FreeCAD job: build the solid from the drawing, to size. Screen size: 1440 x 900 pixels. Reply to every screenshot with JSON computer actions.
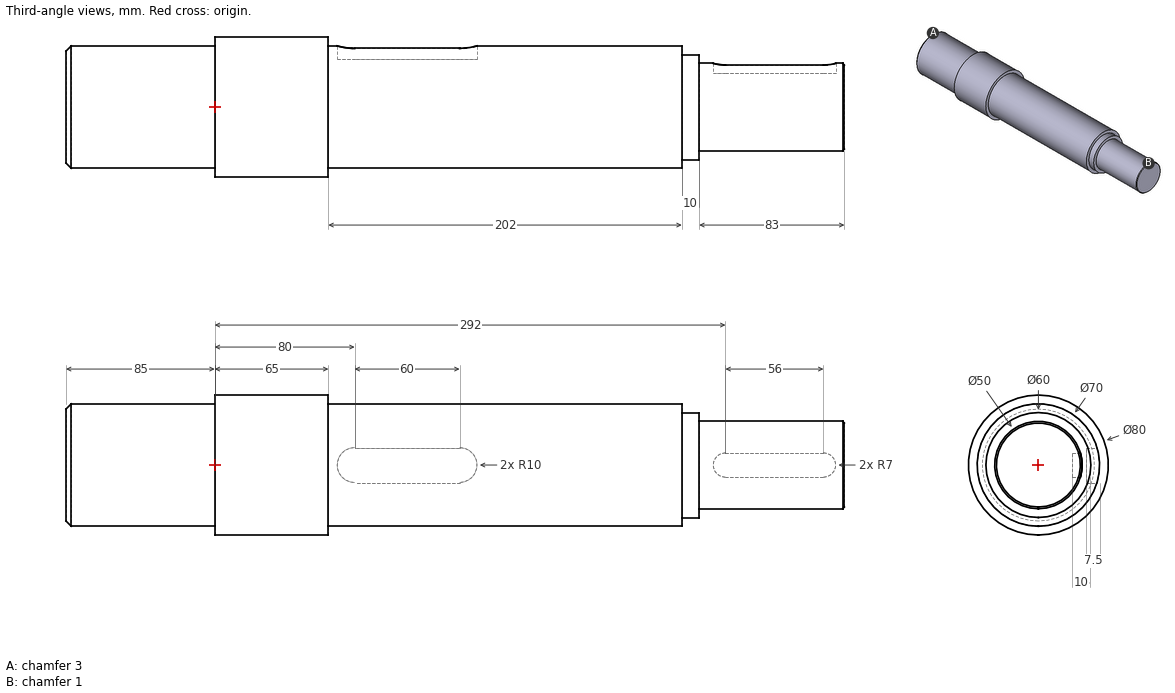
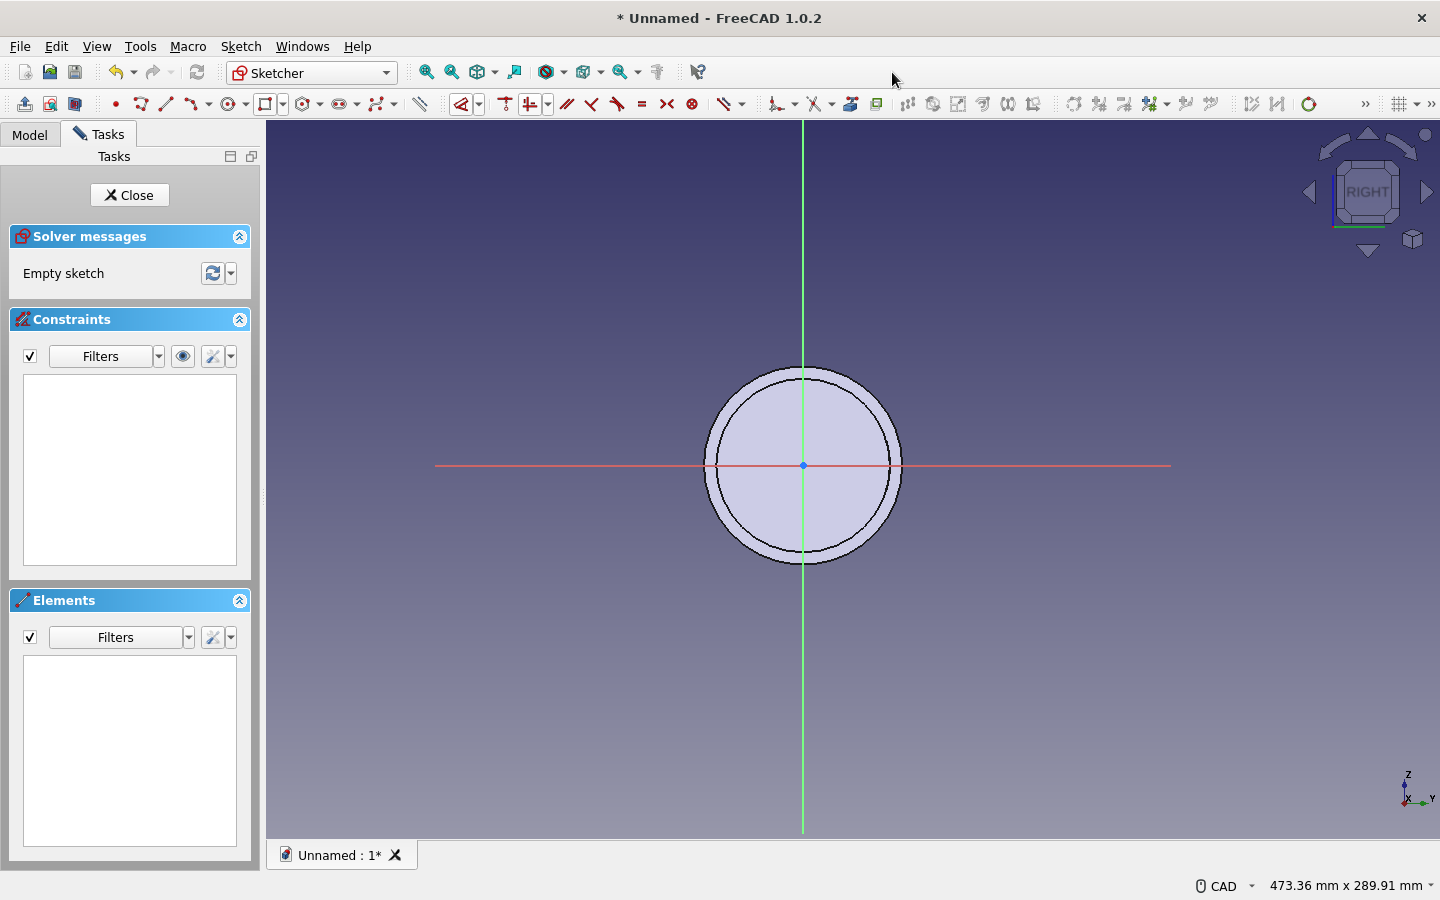
{"action": "scroll", "coordinate": [811, 460], "scroll_direction": "up", "scroll_amount": 6}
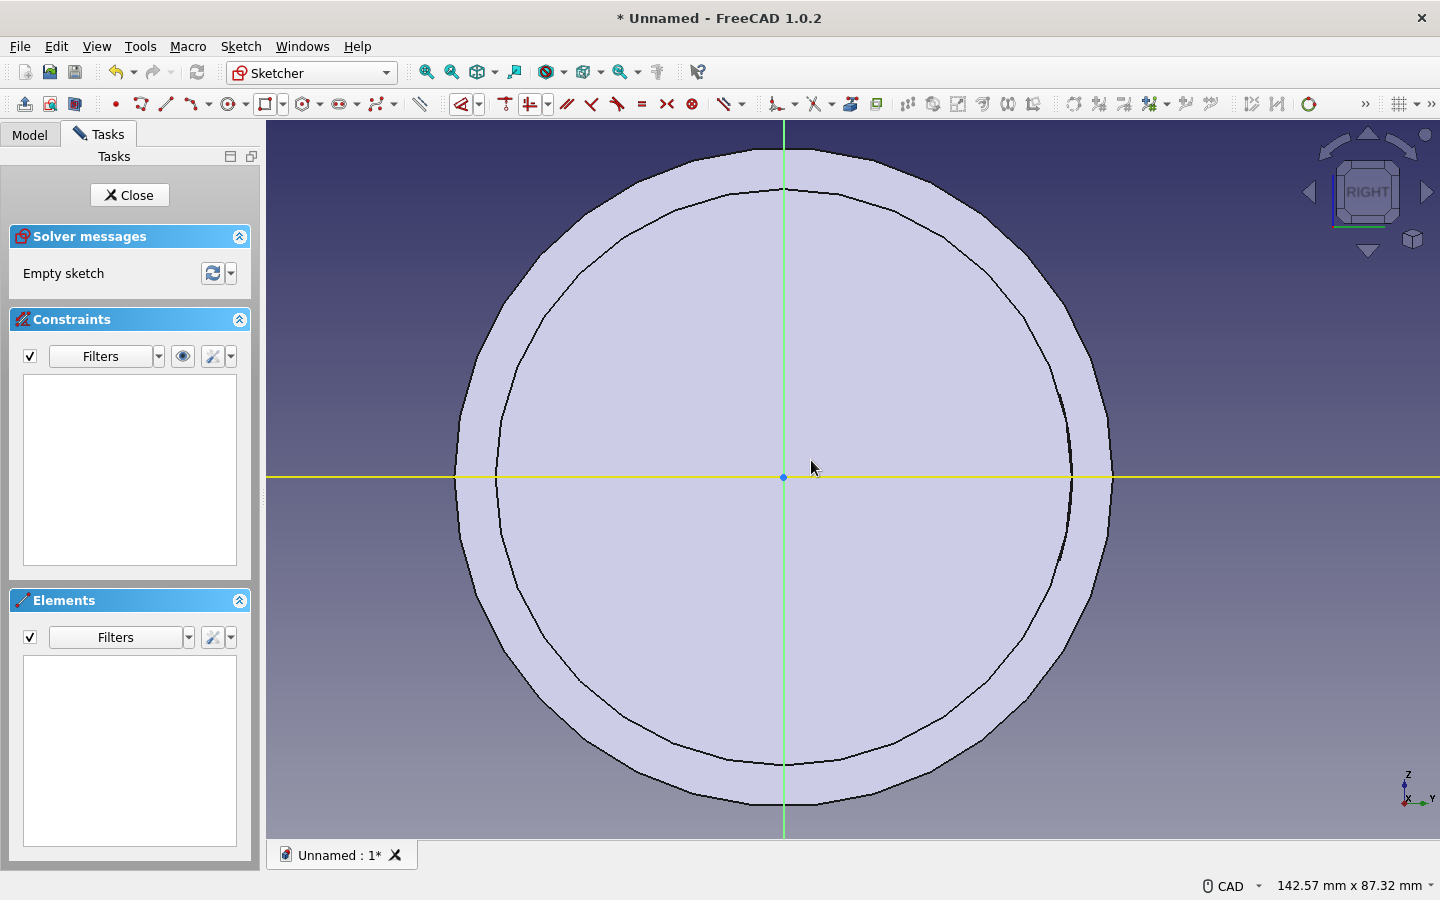
{"action": "key", "text": "g c"}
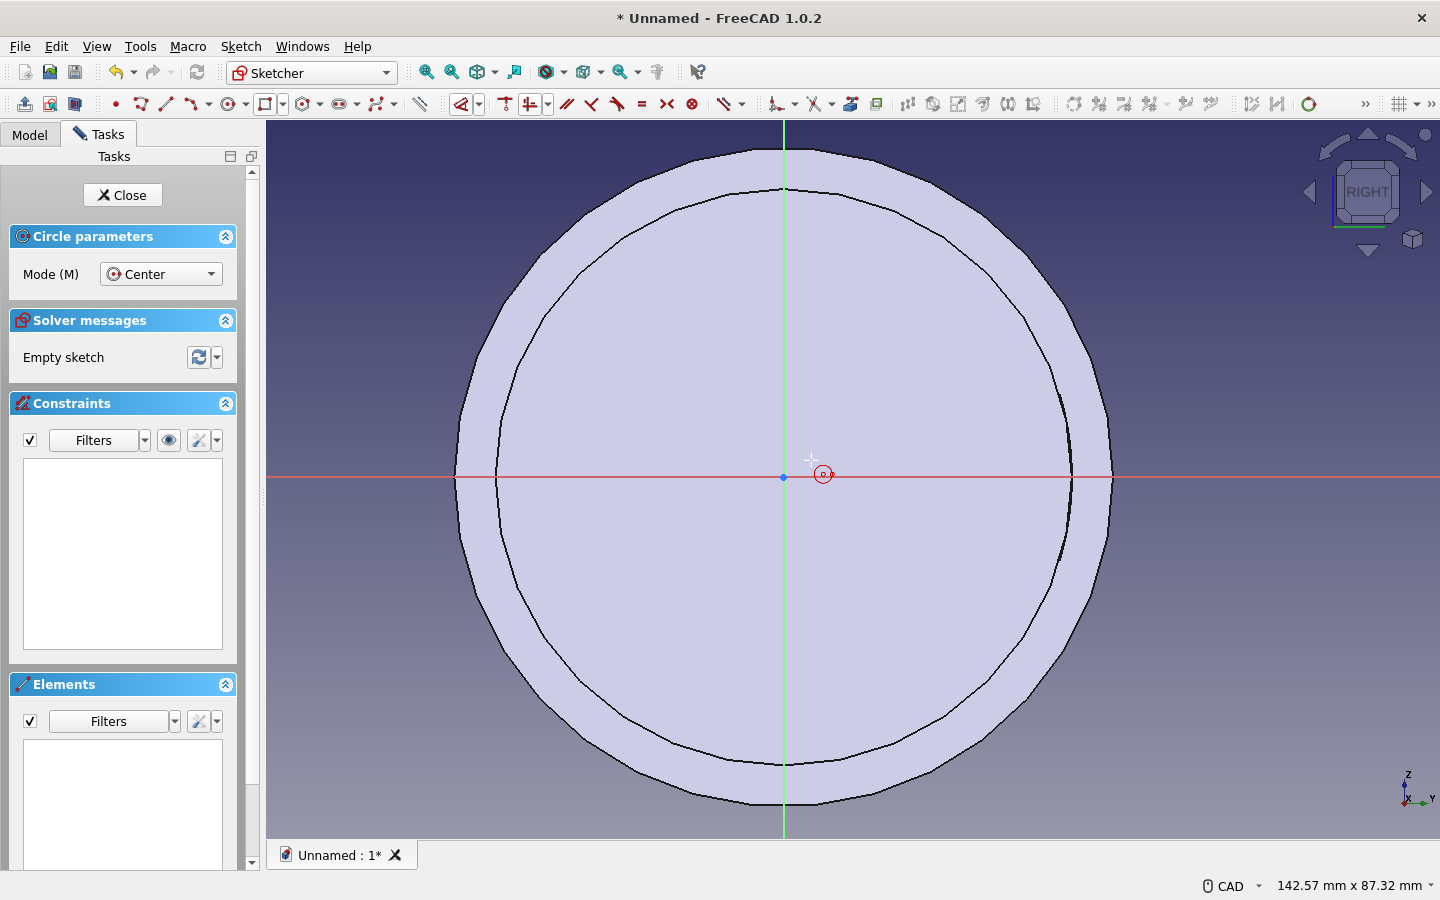
{"action": "left_click", "coordinate": [784, 477]}
{"action": "left_click", "coordinate": [958, 303]}
{"action": "key", "text": "Escape"}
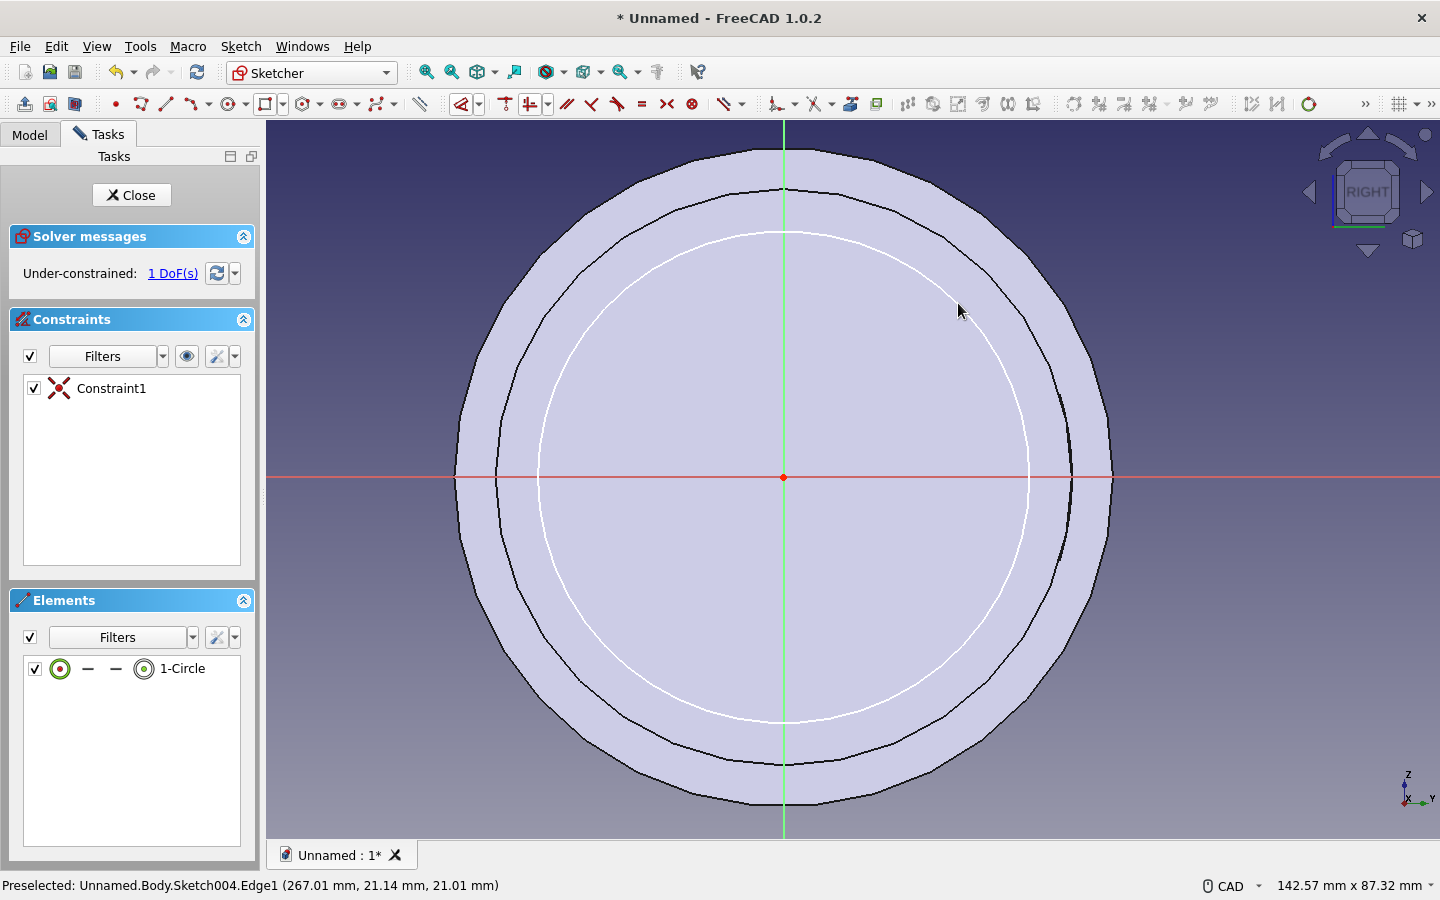
{"action": "left_click", "coordinate": [460, 104]}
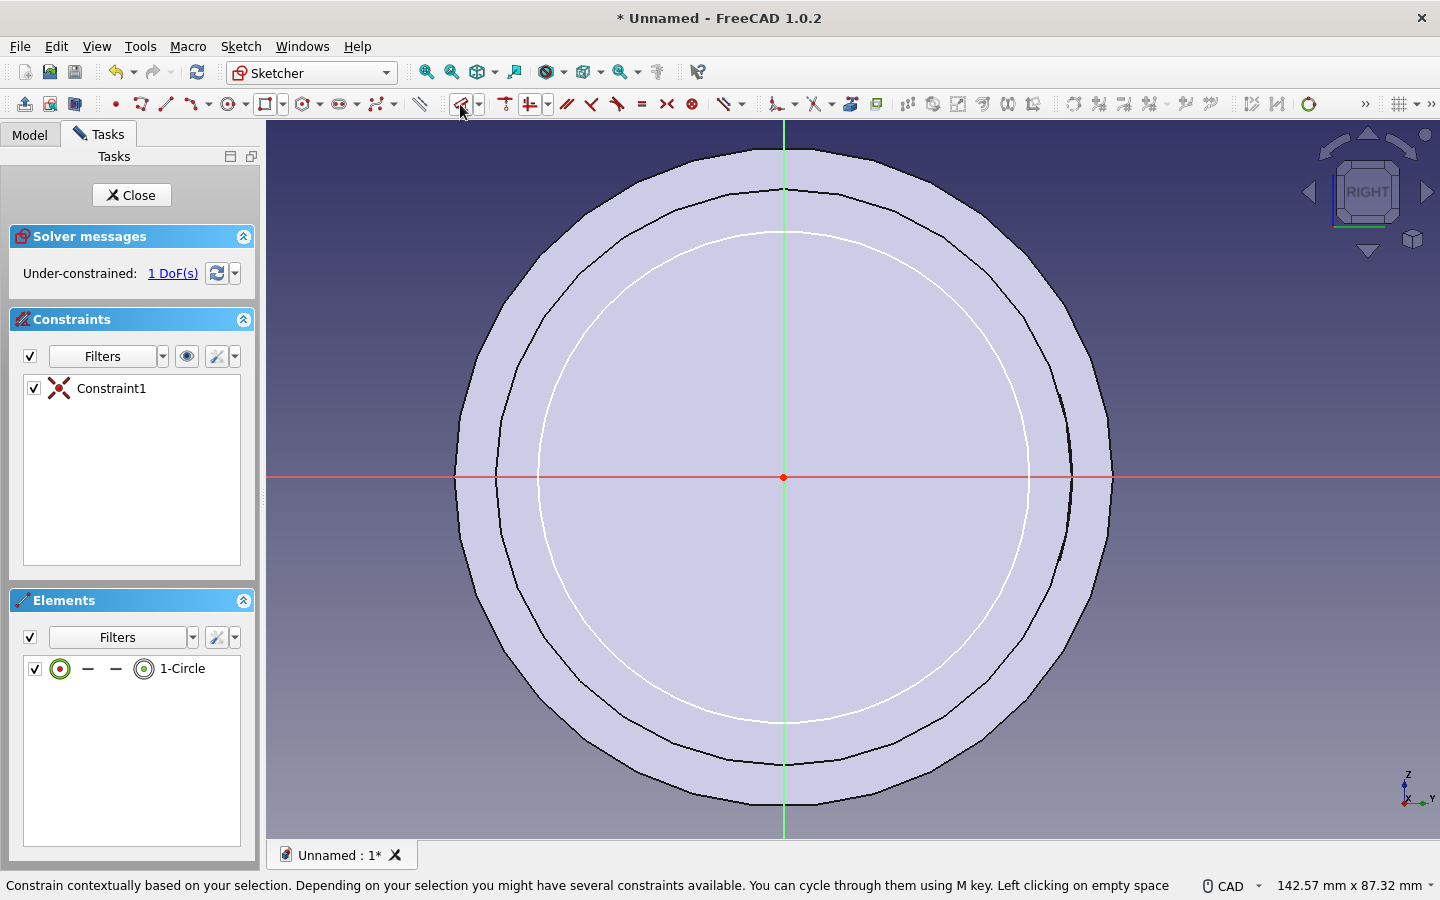
{"action": "left_click", "coordinate": [957, 303]}
{"action": "left_click", "coordinate": [980, 280]}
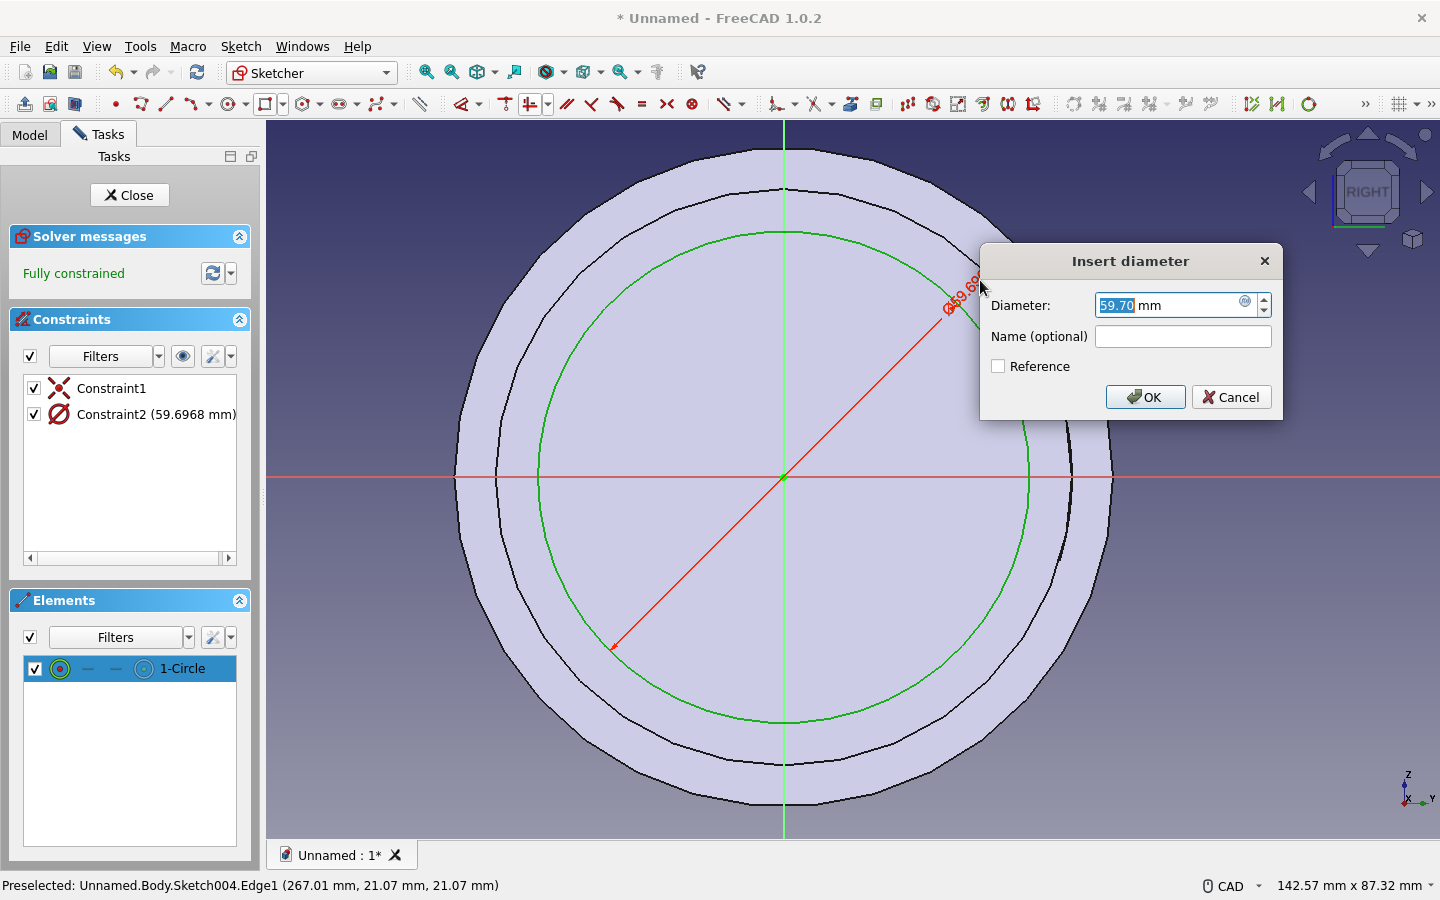
{"action": "type", "text": "60"}
{"action": "key", "text": "Return"}
{"action": "key", "text": "Escape"}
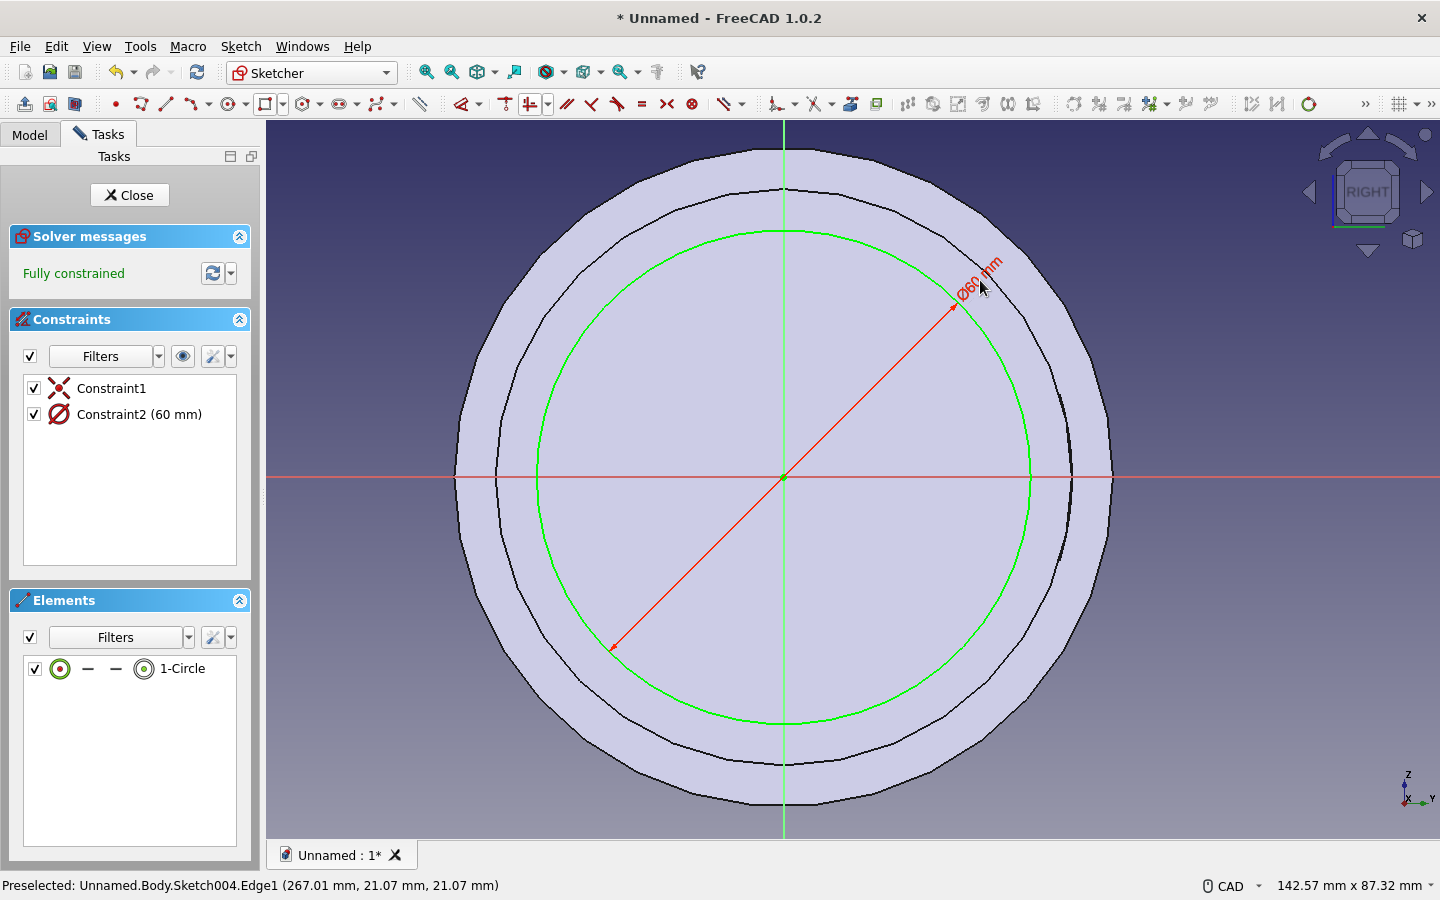
{"action": "left_click", "coordinate": [130, 195]}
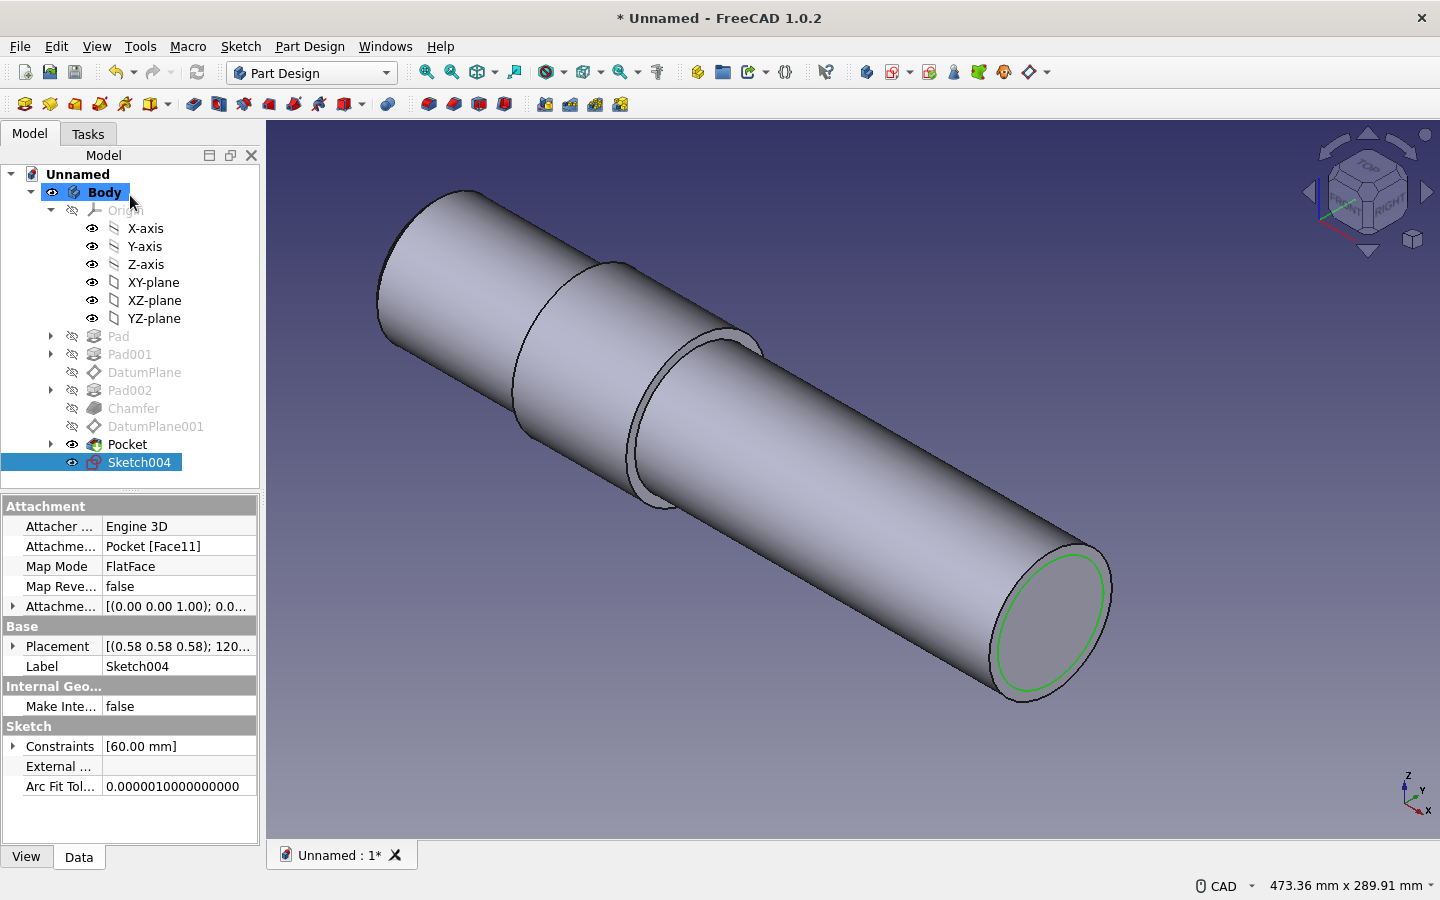
{"action": "left_click", "coordinate": [25, 104]}